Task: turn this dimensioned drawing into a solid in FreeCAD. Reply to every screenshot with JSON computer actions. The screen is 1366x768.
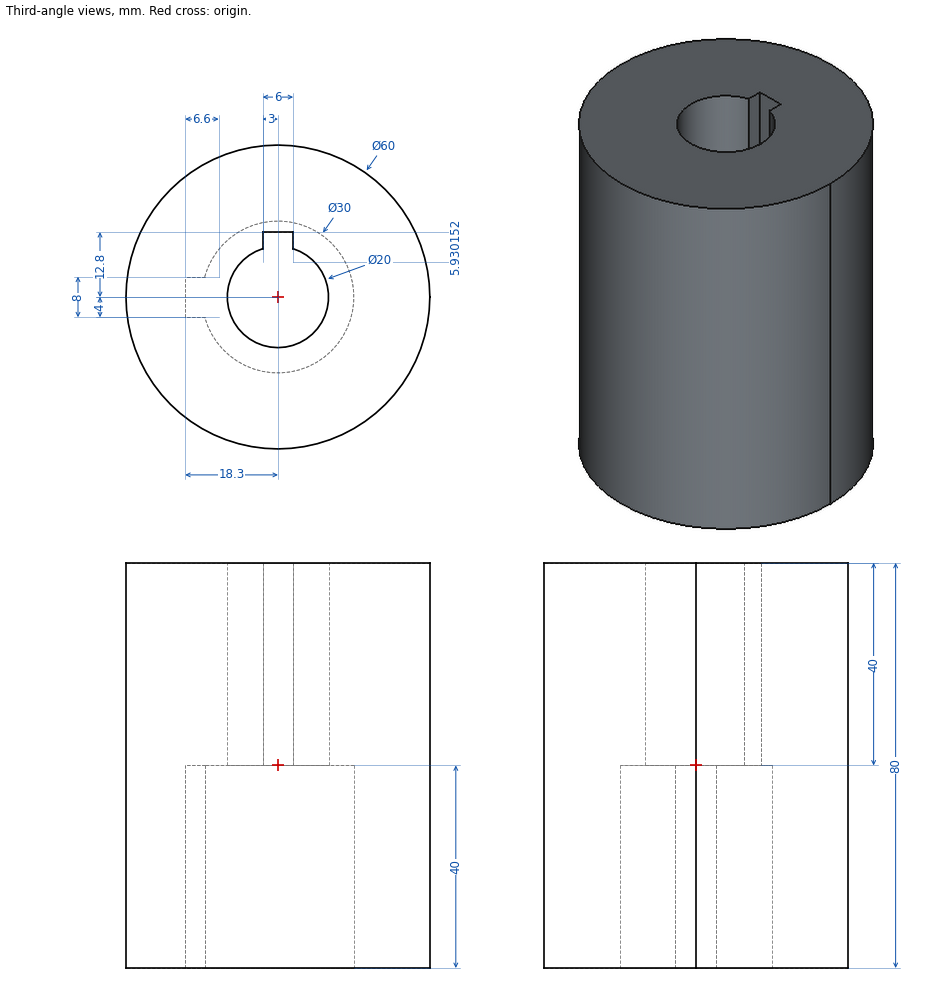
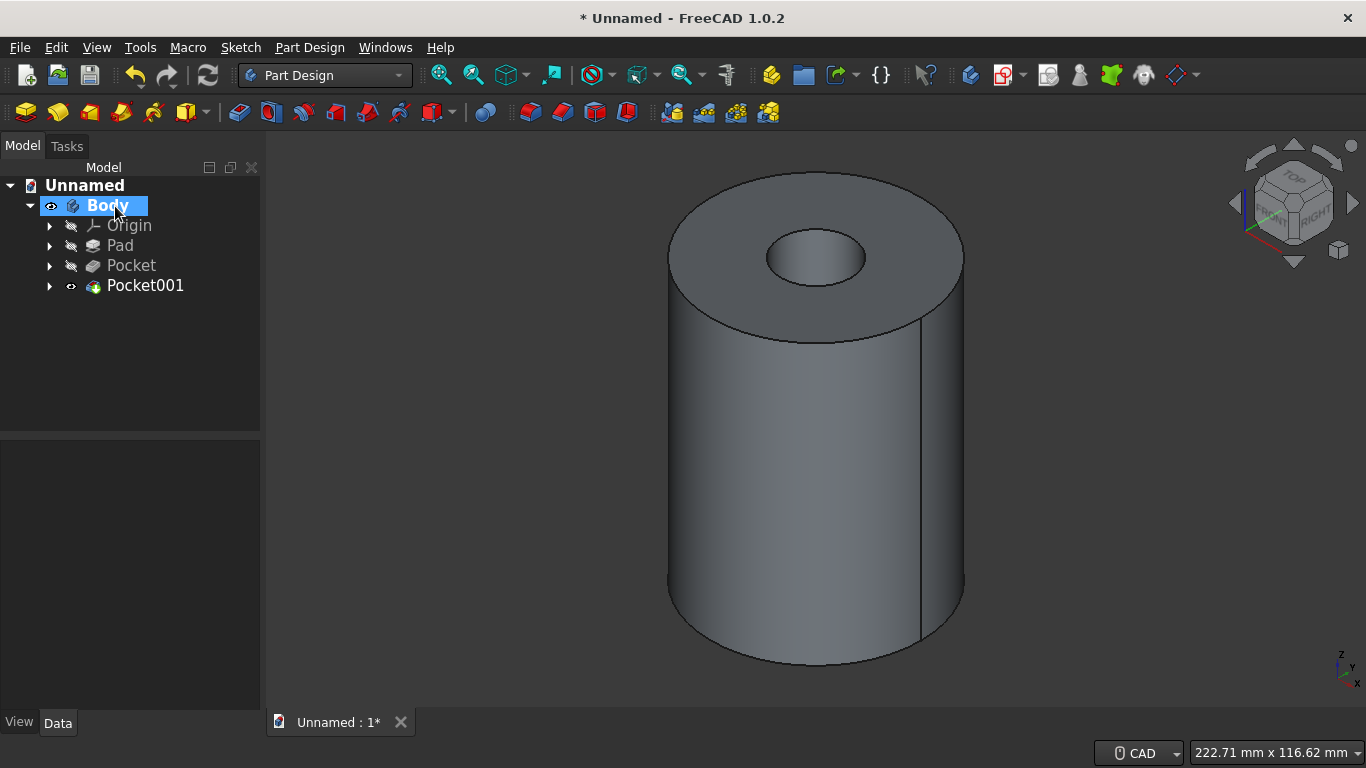
{"action": "left_click", "coordinate": [846, 205]}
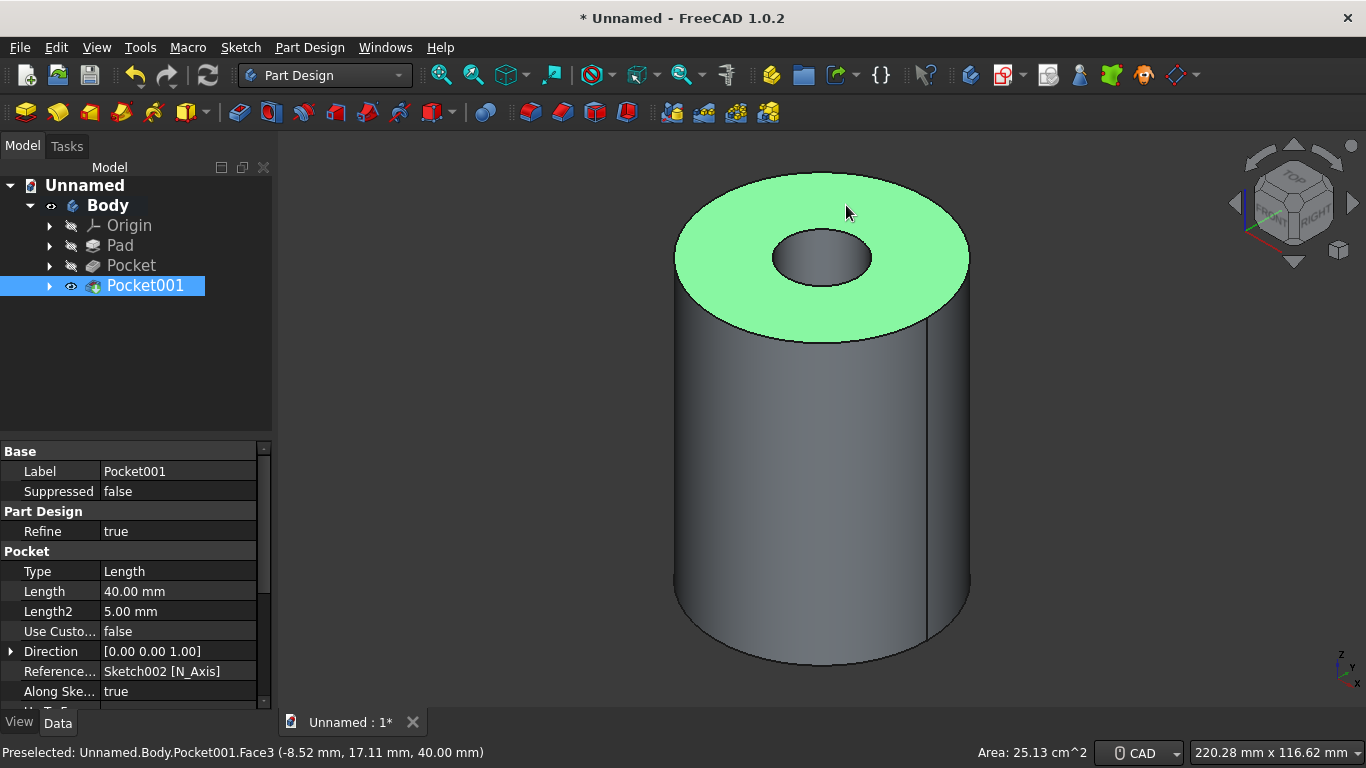
{"action": "left_click", "coordinate": [1004, 76]}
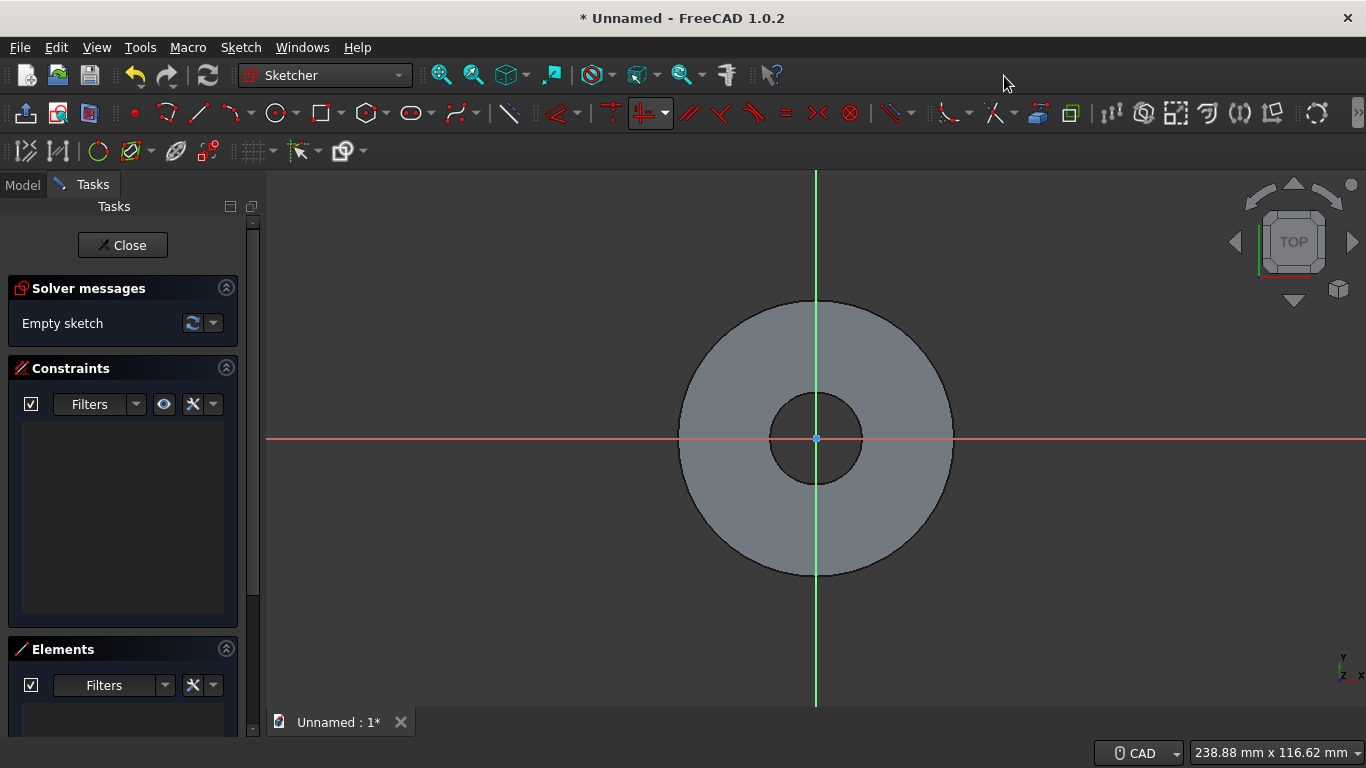
{"action": "scroll", "coordinate": [830, 403], "scroll_direction": "up", "scroll_amount": 9}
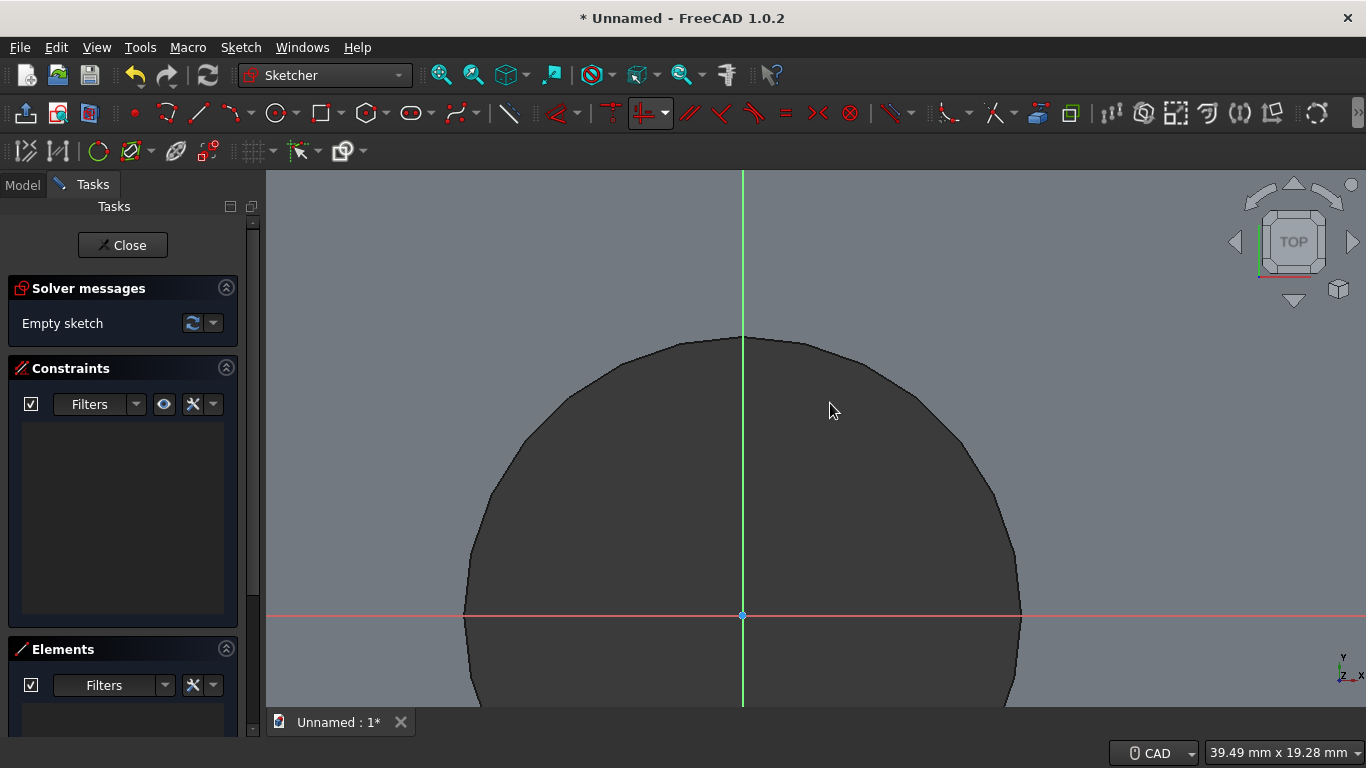
{"action": "key", "text": "g r"}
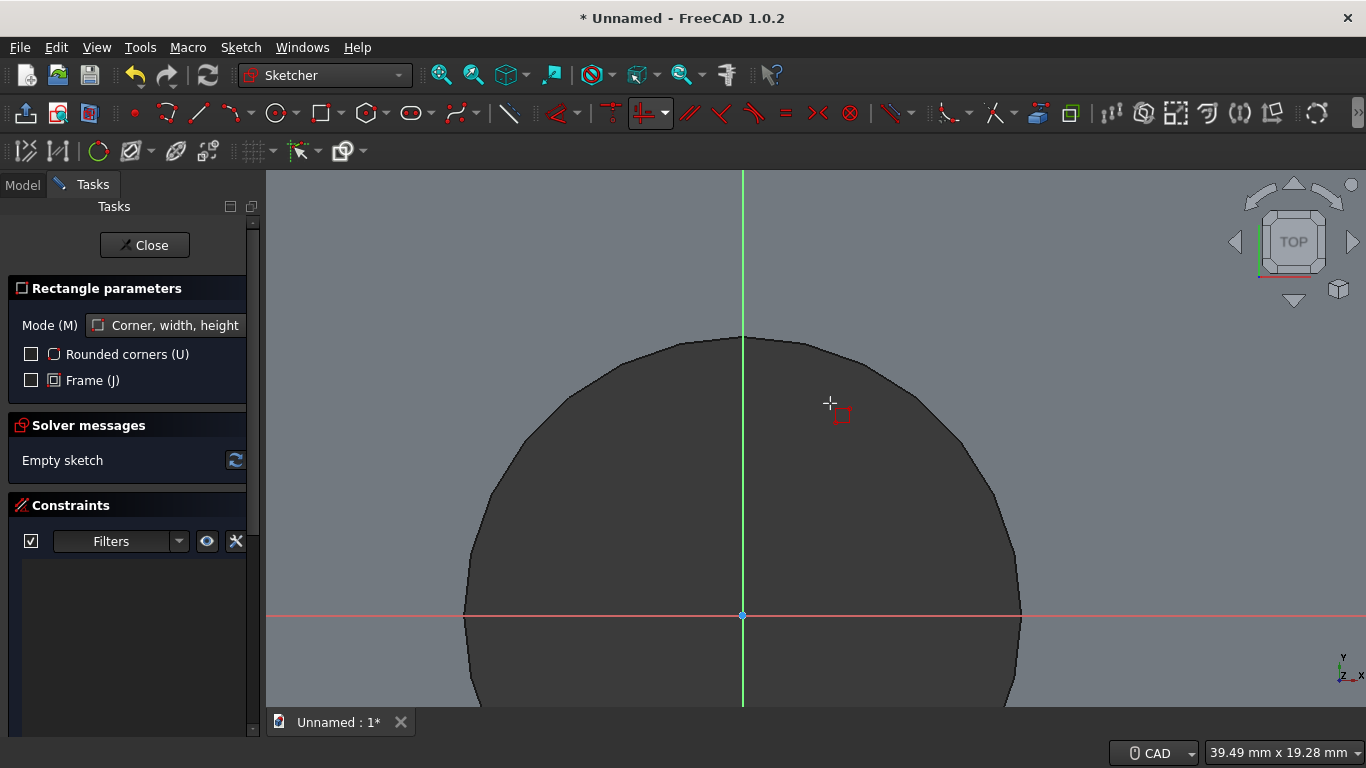
{"action": "left_click", "coordinate": [659, 259]}
{"action": "mouse_move", "coordinate": [826, 424]}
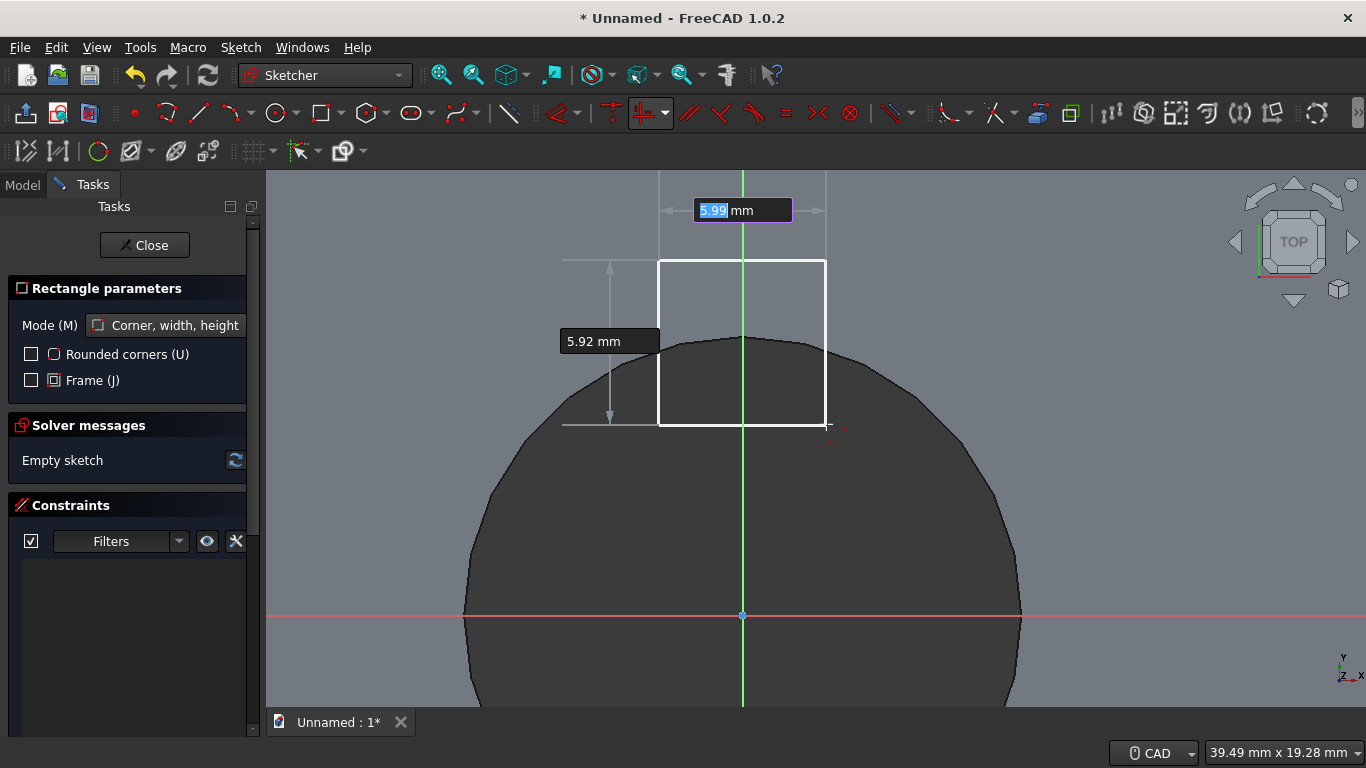
{"action": "type", "text": "6"}
{"action": "key", "text": "Tab"}
{"action": "type", "text": "5.930152"}
{"action": "key", "text": "Return"}
{"action": "key", "text": "Escape"}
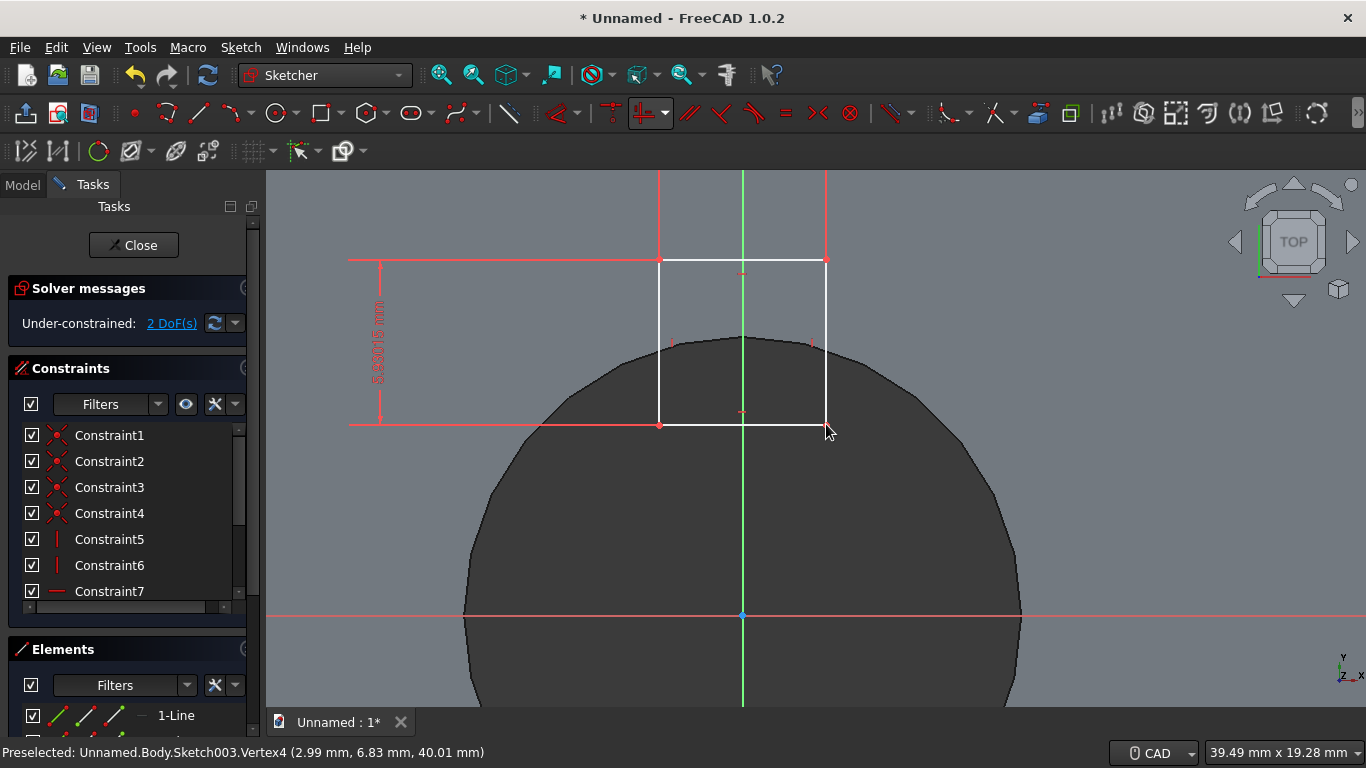
{"action": "left_click", "coordinate": [556, 114]}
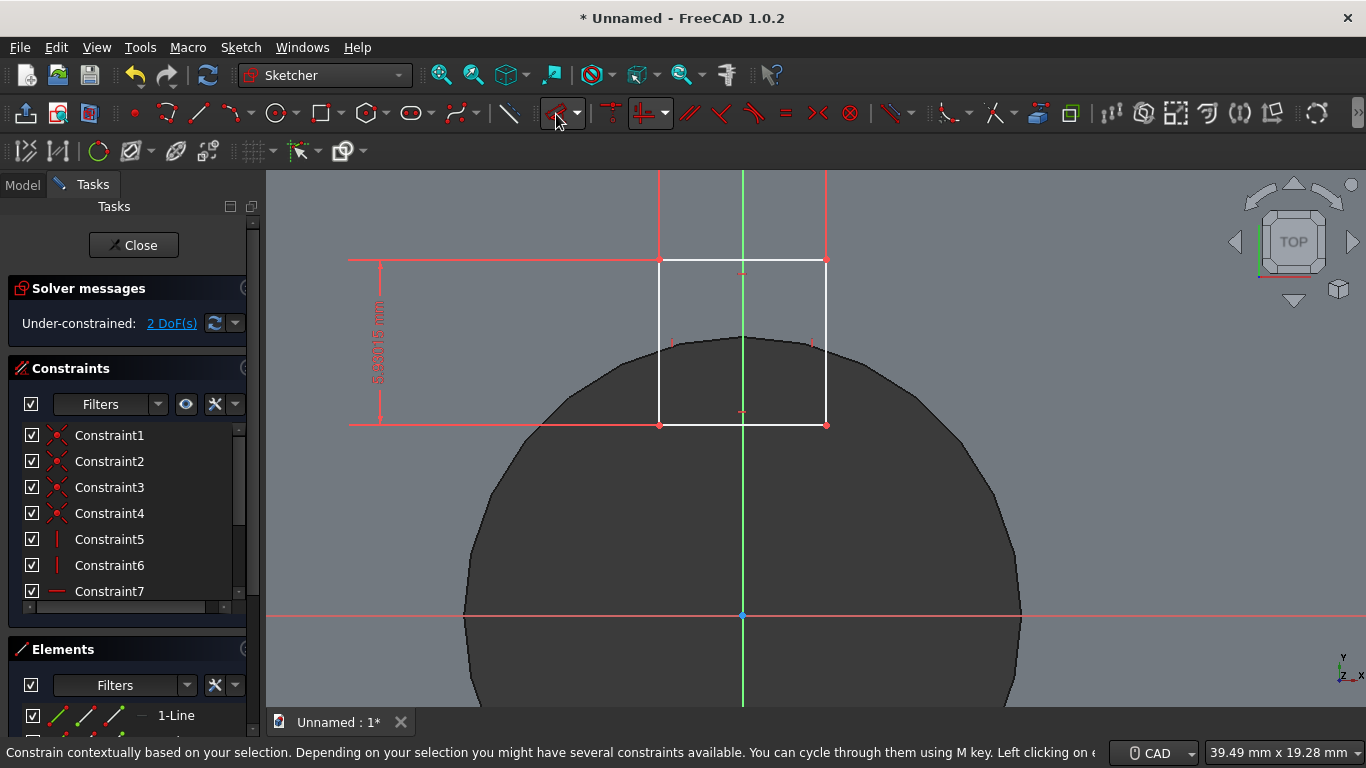
{"action": "left_click", "coordinate": [659, 260]}
{"action": "left_click", "coordinate": [701, 650]}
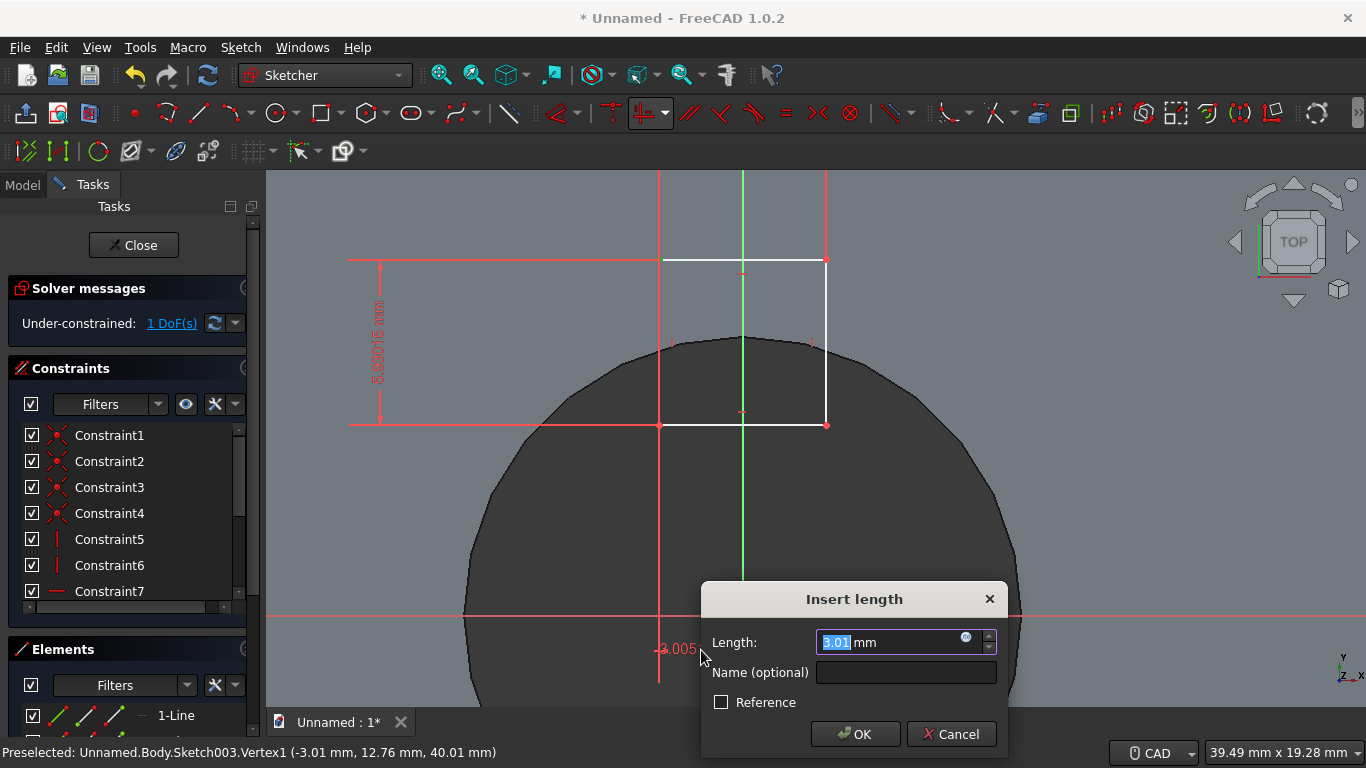
{"action": "type", "text": "3"}
{"action": "key", "text": "Return"}